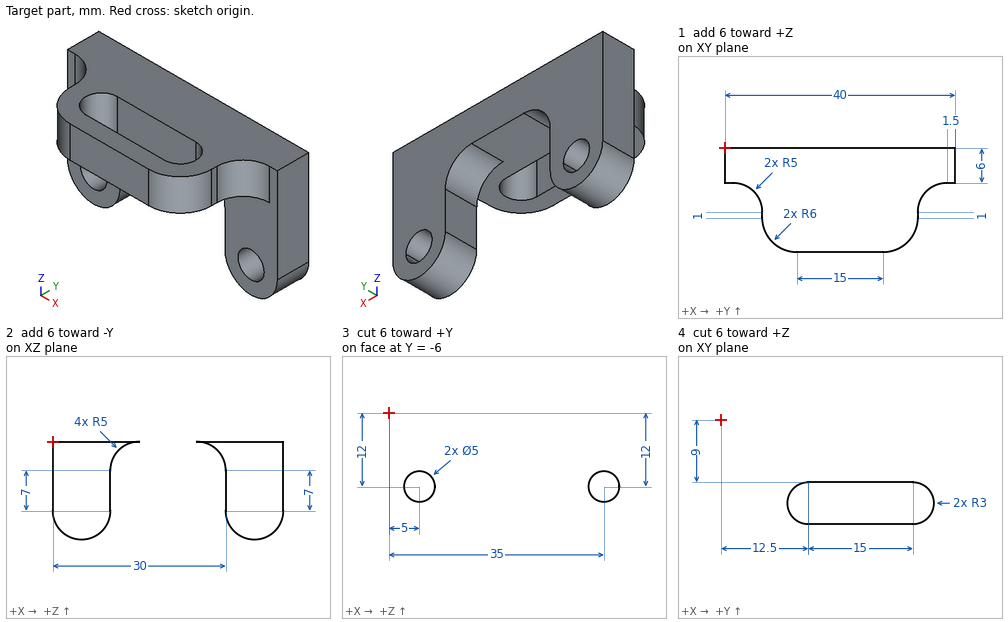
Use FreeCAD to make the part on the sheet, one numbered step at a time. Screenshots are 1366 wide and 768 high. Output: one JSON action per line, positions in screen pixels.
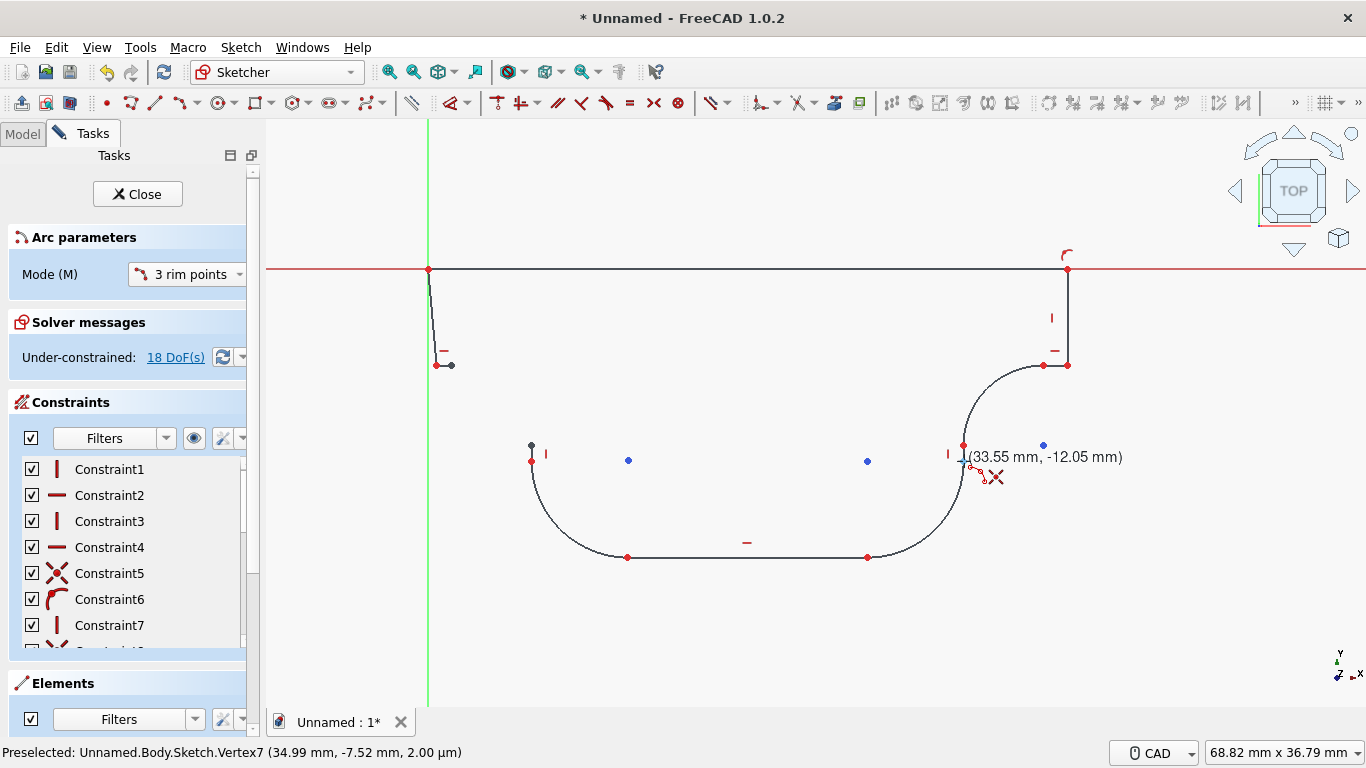
{"action": "scroll", "coordinate": [452, 365], "scroll_direction": "up", "scroll_amount": 2}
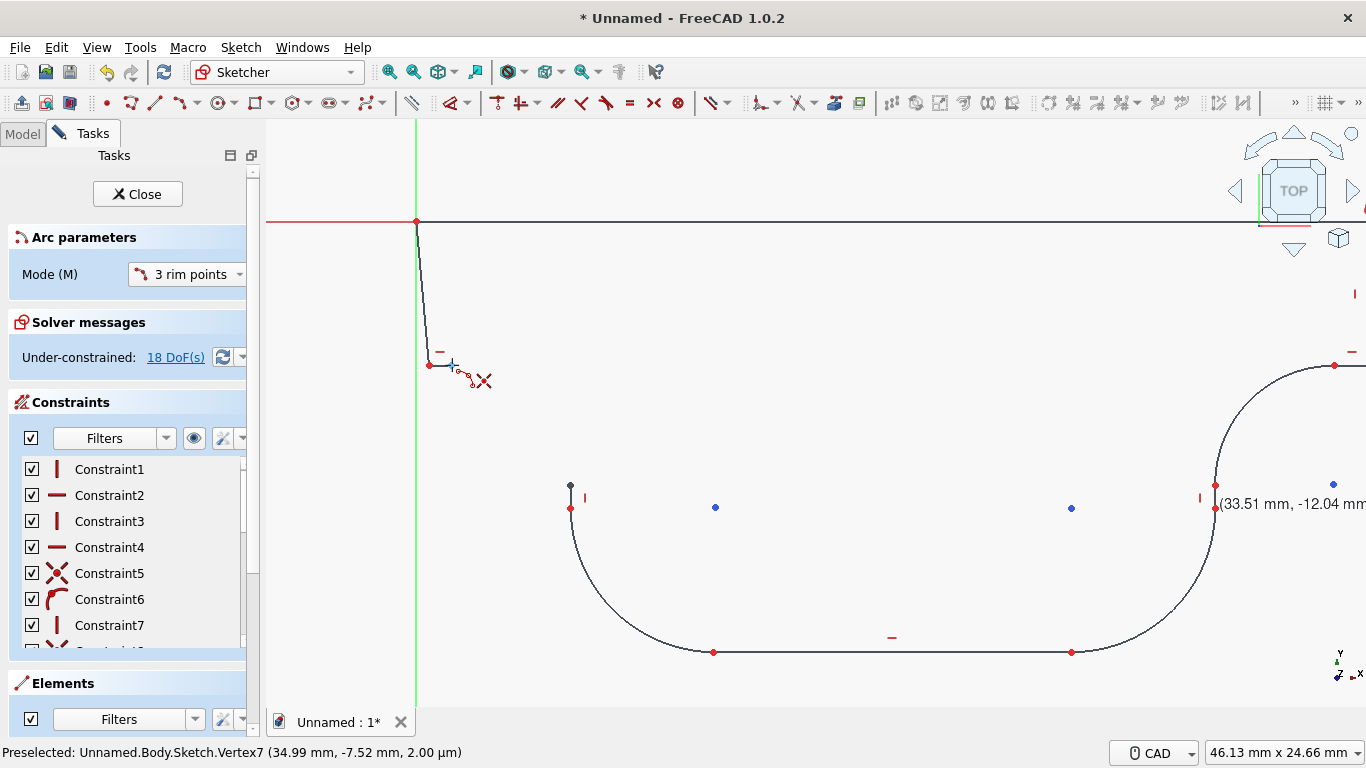
{"action": "left_click", "coordinate": [451, 366]}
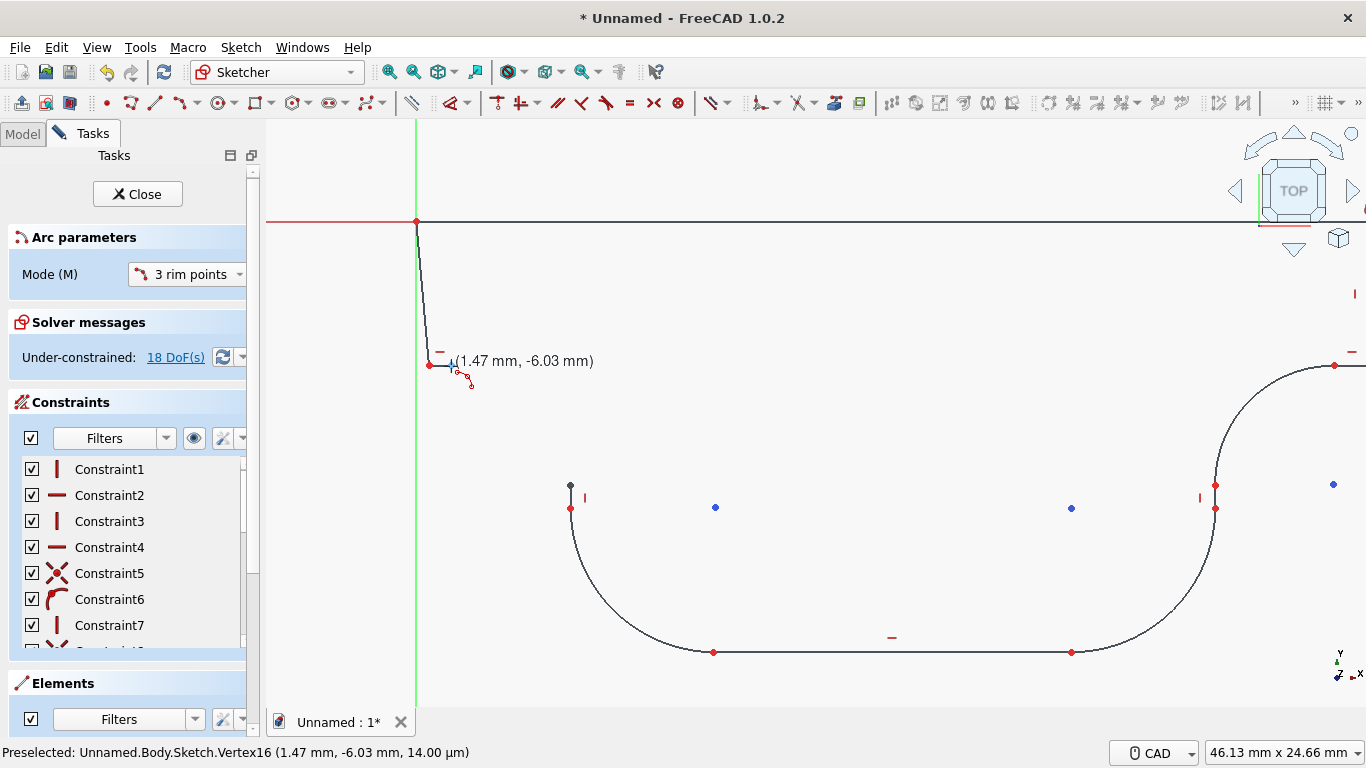
{"action": "scroll", "coordinate": [571, 484], "scroll_direction": "up", "scroll_amount": 2}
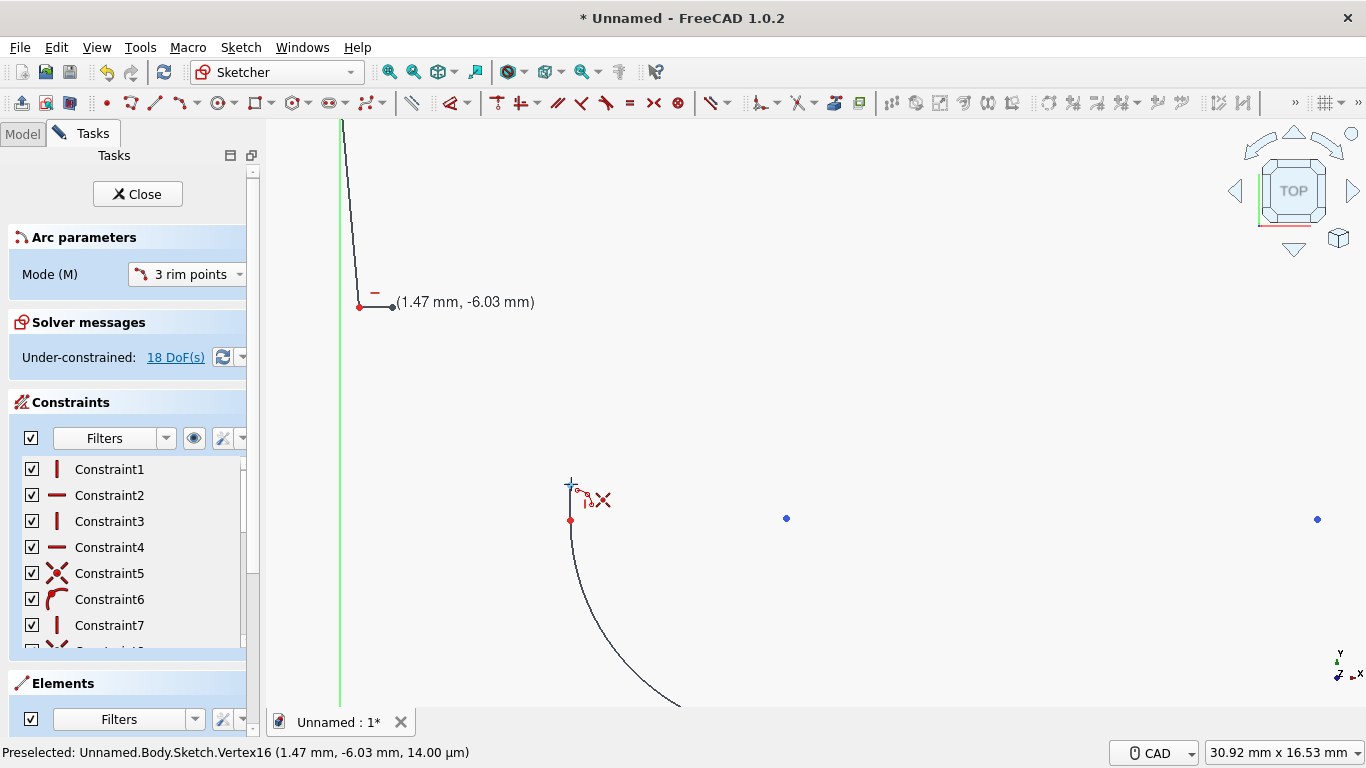
{"action": "left_click", "coordinate": [570, 485]}
{"action": "left_click", "coordinate": [519, 358]}
{"action": "key", "text": "Escape"}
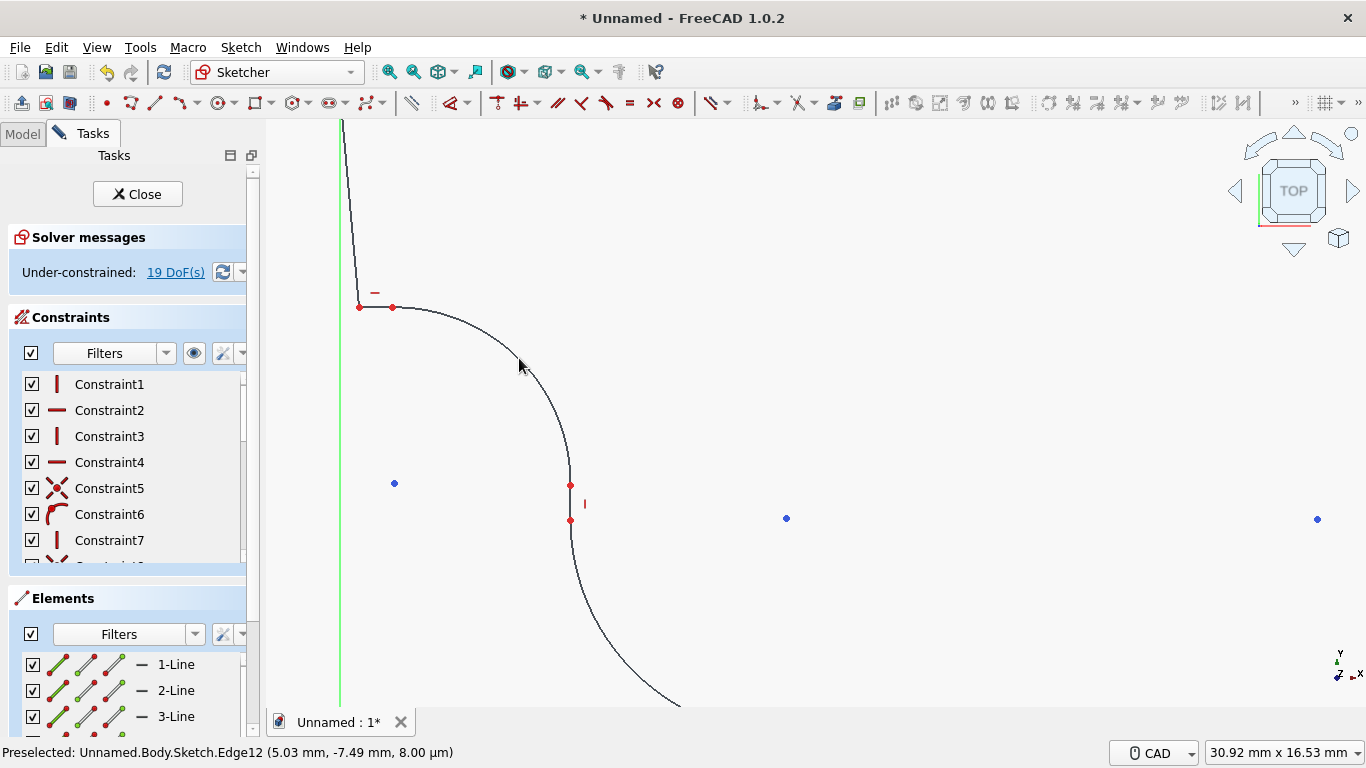
{"action": "scroll", "coordinate": [570, 496], "scroll_direction": "up", "scroll_amount": 2}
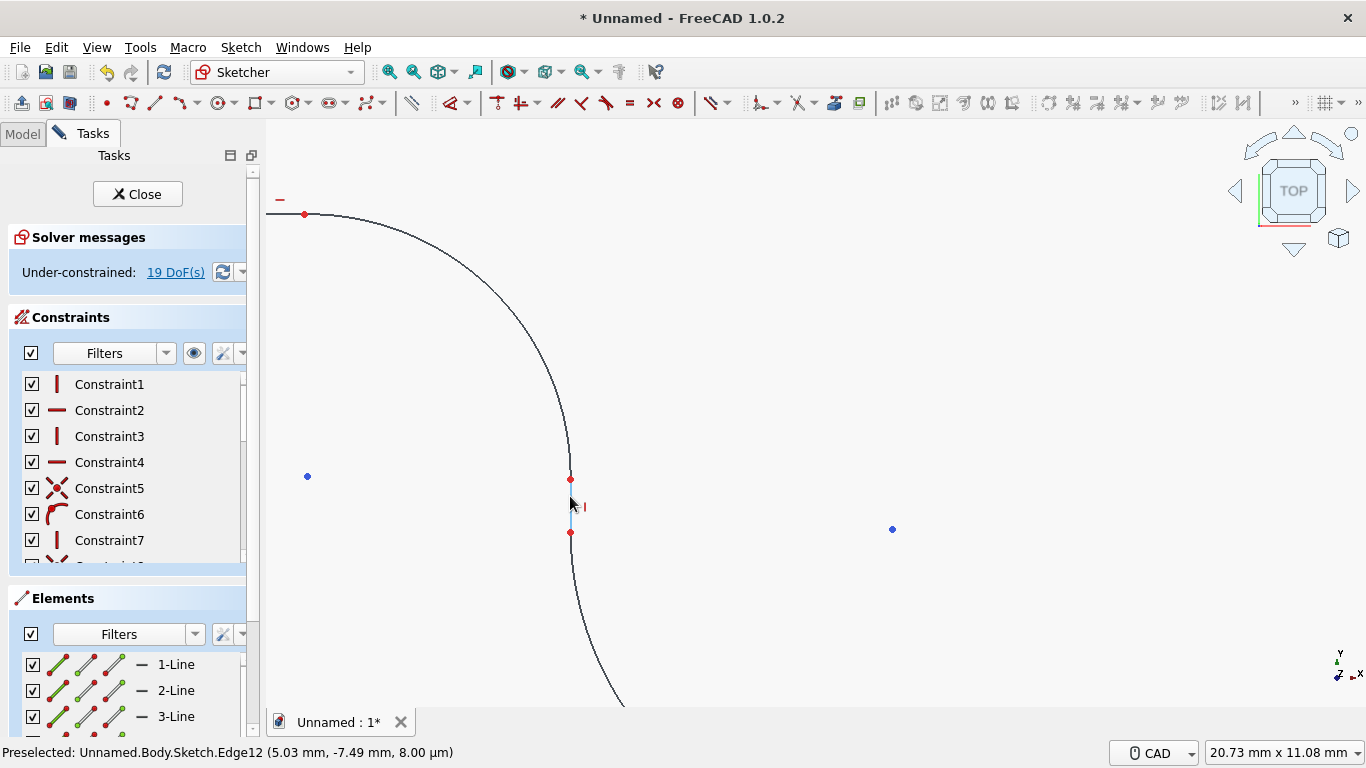
{"action": "left_click", "coordinate": [571, 496]}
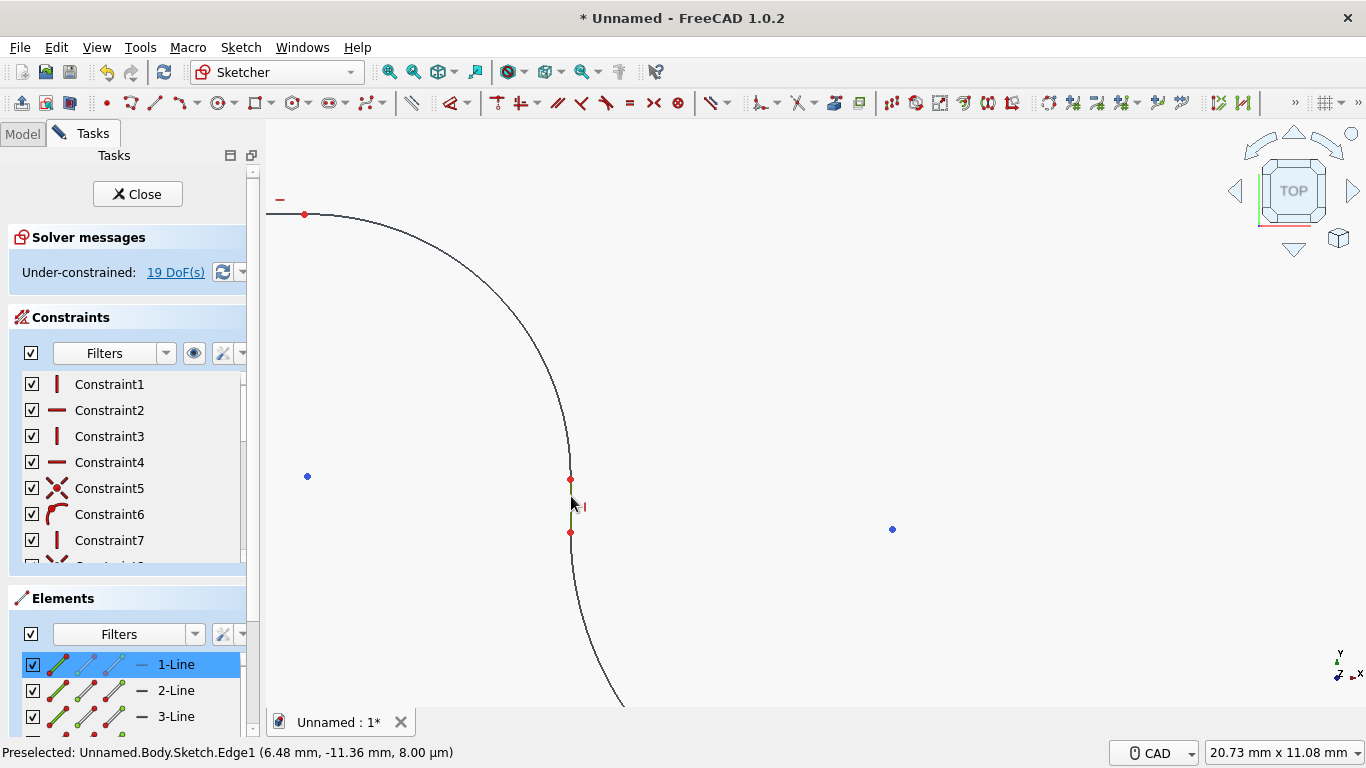
{"action": "left_click", "coordinate": [606, 677]}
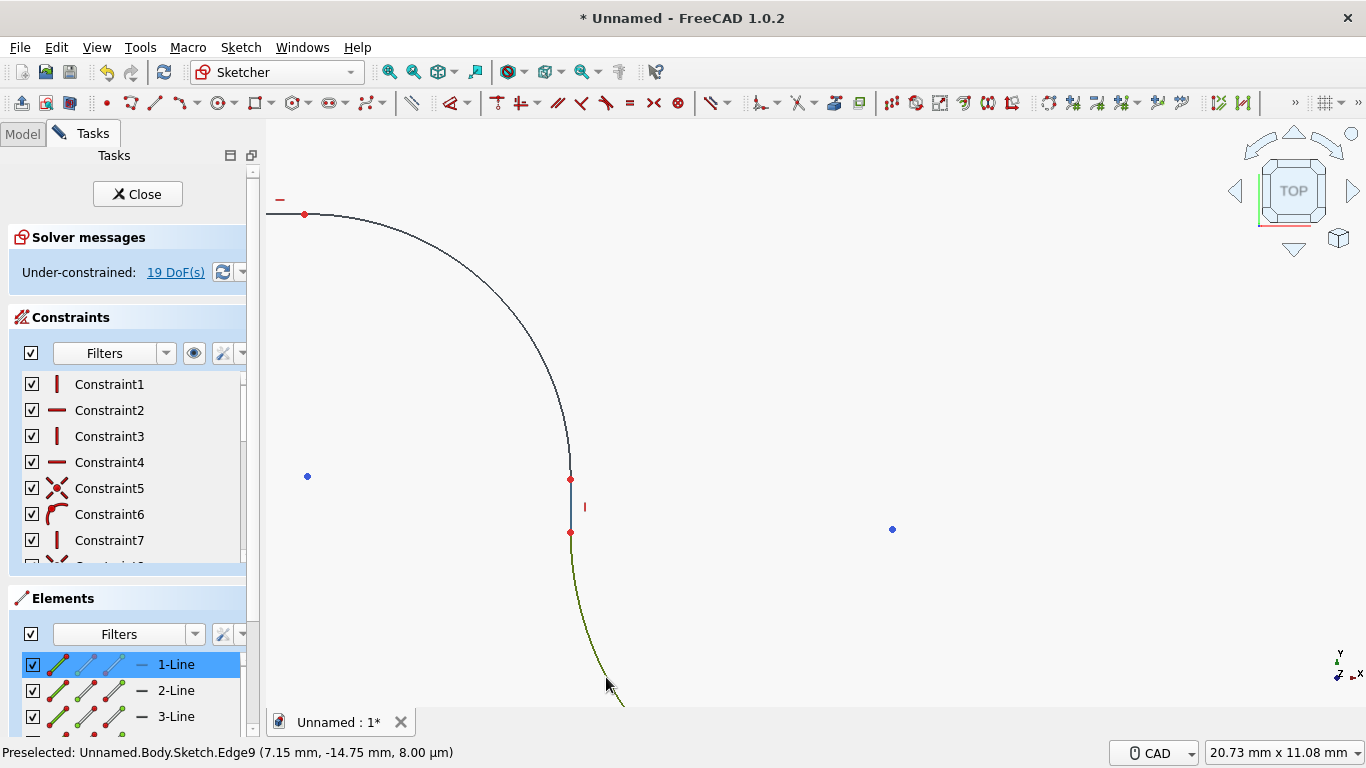
{"action": "key", "text": "t"}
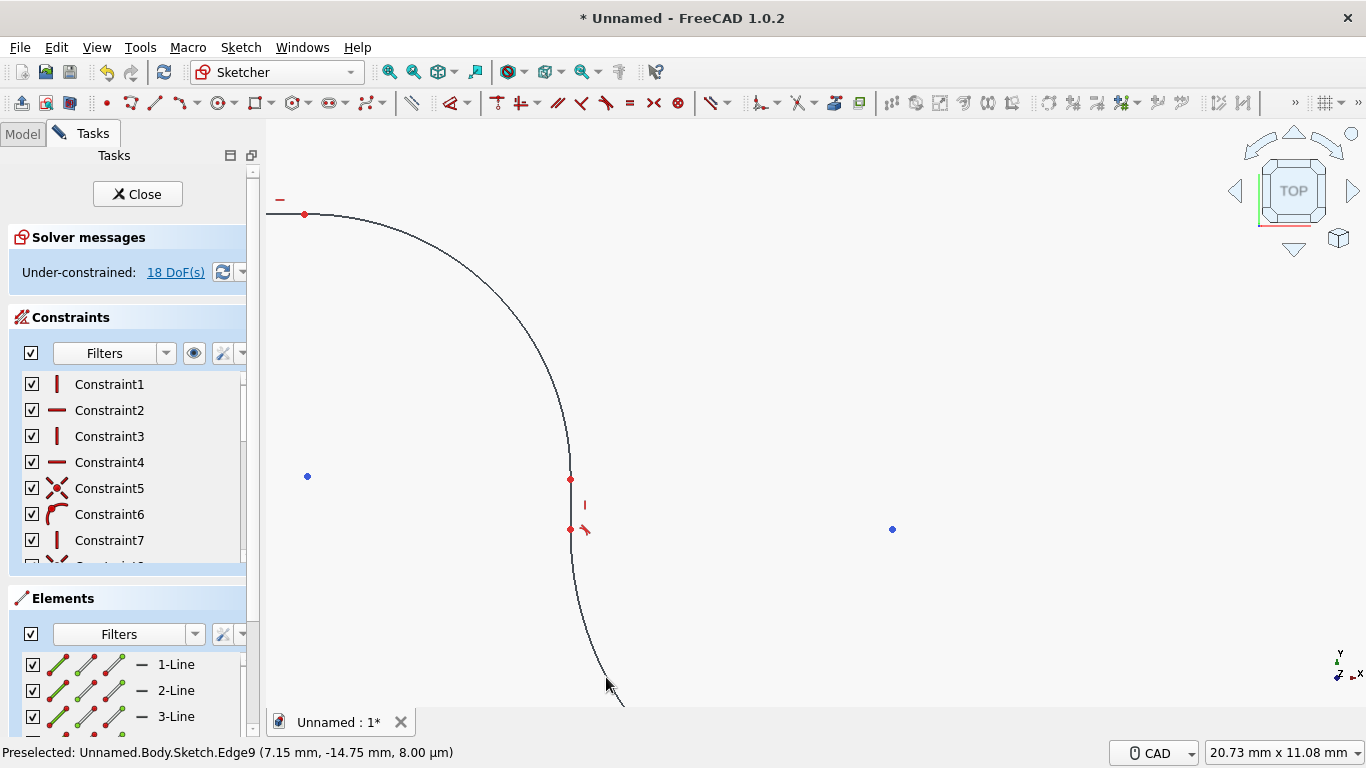
{"action": "left_click", "coordinate": [571, 495]}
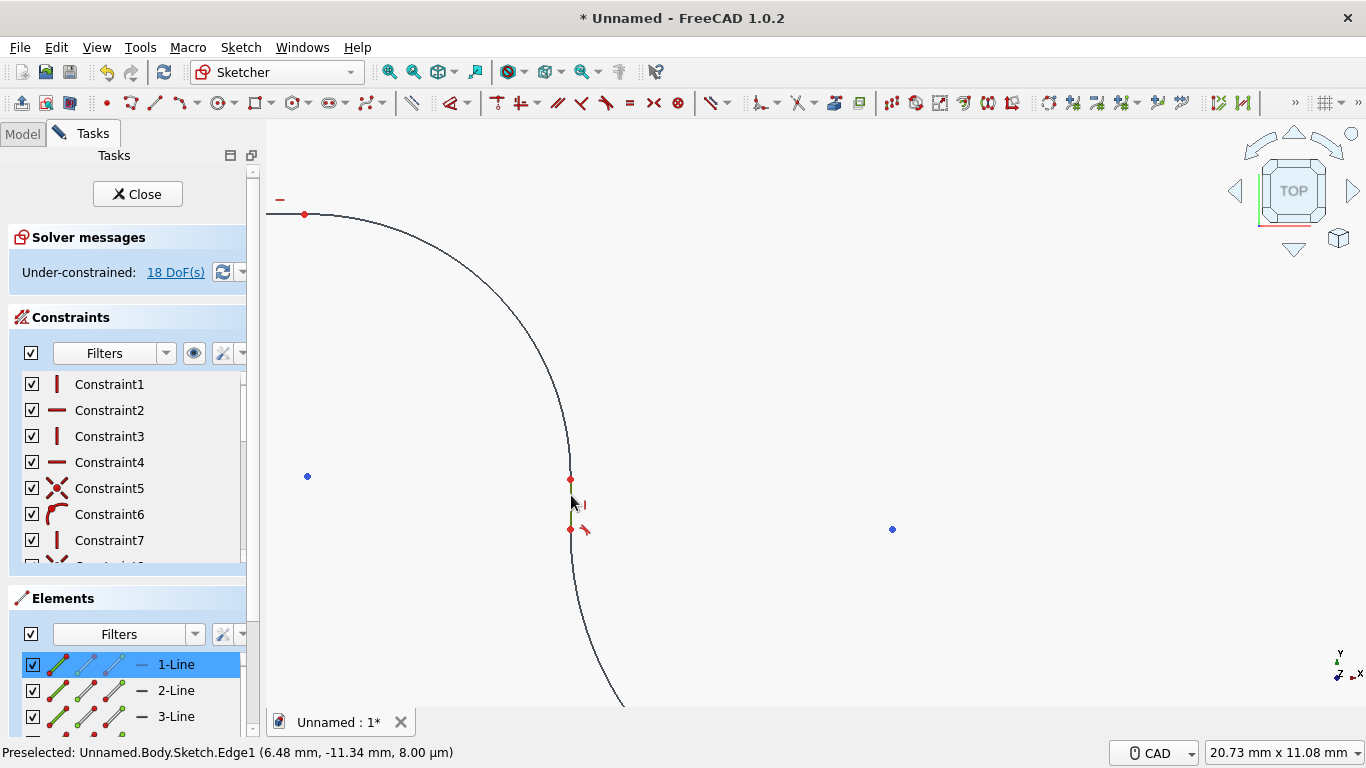
{"action": "left_click", "coordinate": [542, 359]}